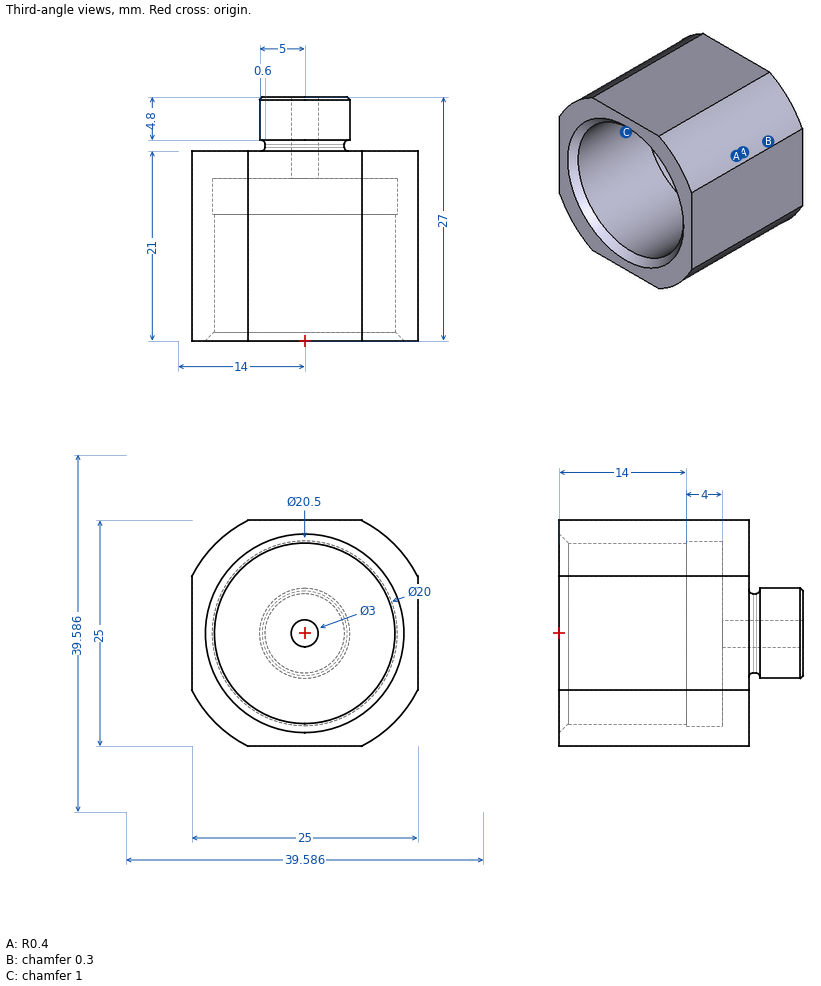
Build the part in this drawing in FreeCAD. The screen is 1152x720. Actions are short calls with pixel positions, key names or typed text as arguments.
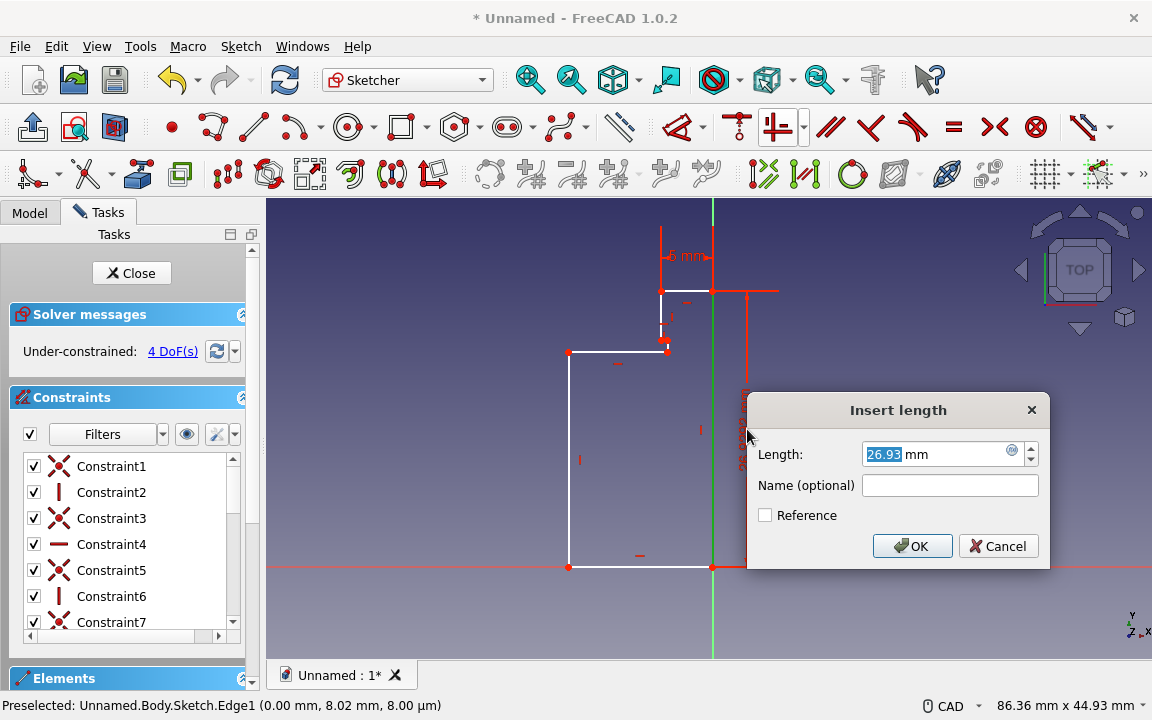
text(27)
key(Return)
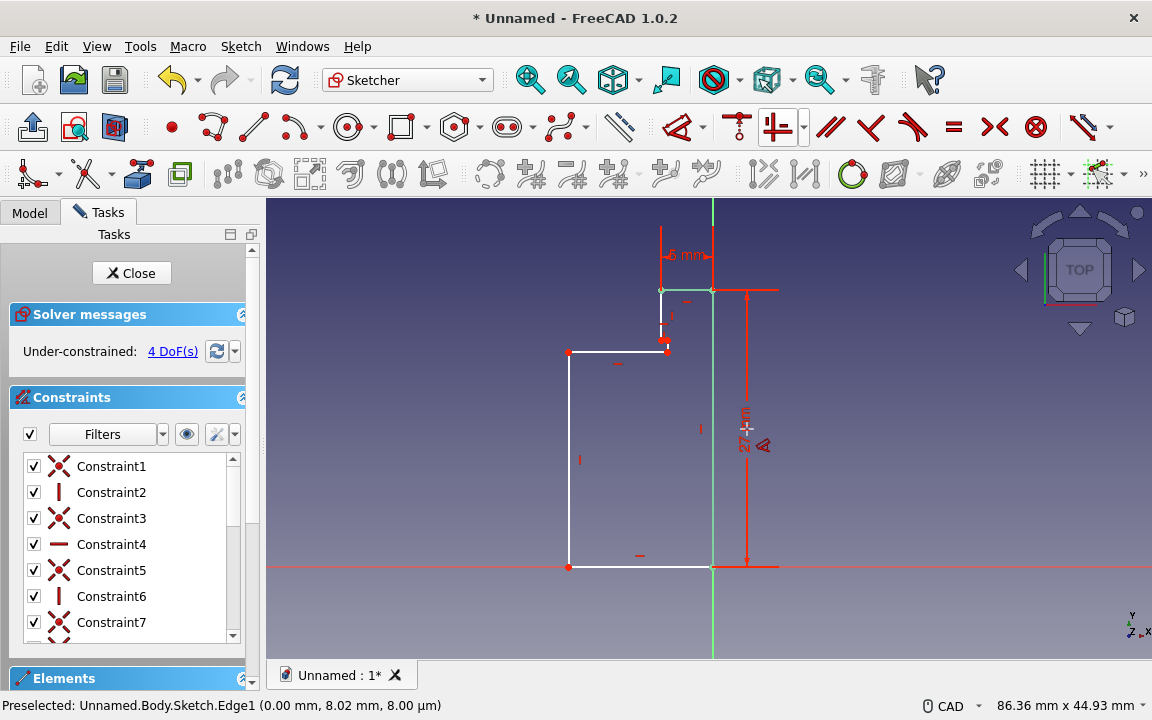
click(569, 417)
click(535, 460)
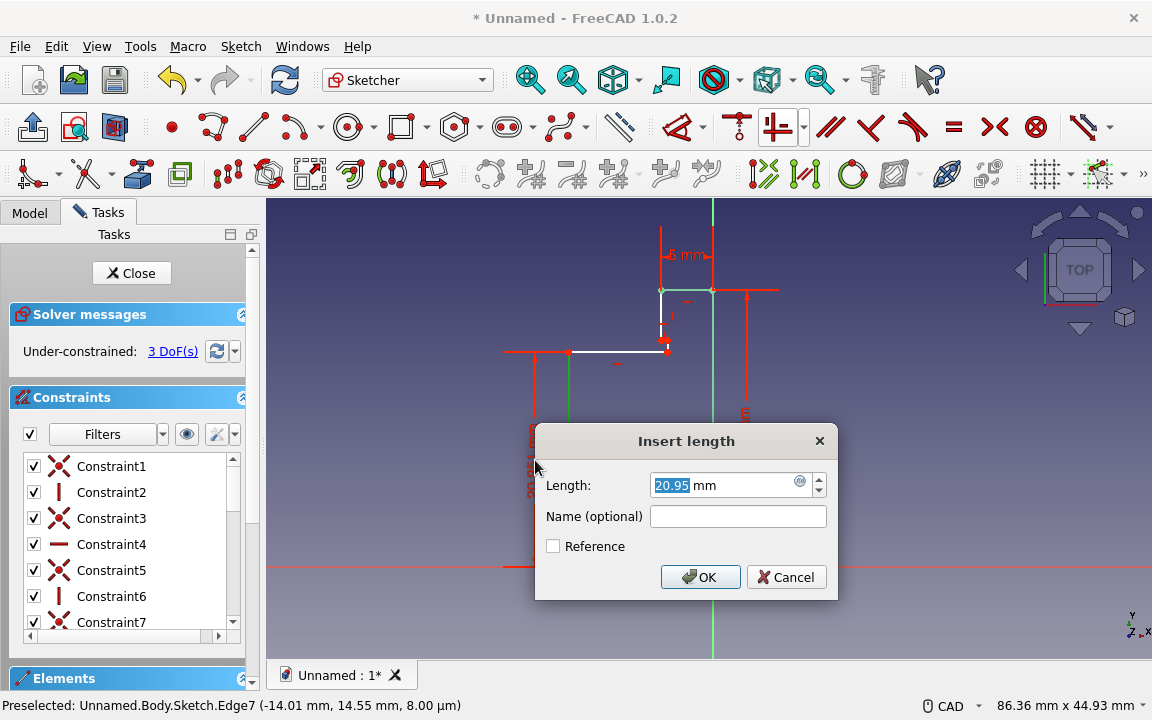
text(21)
key(Return)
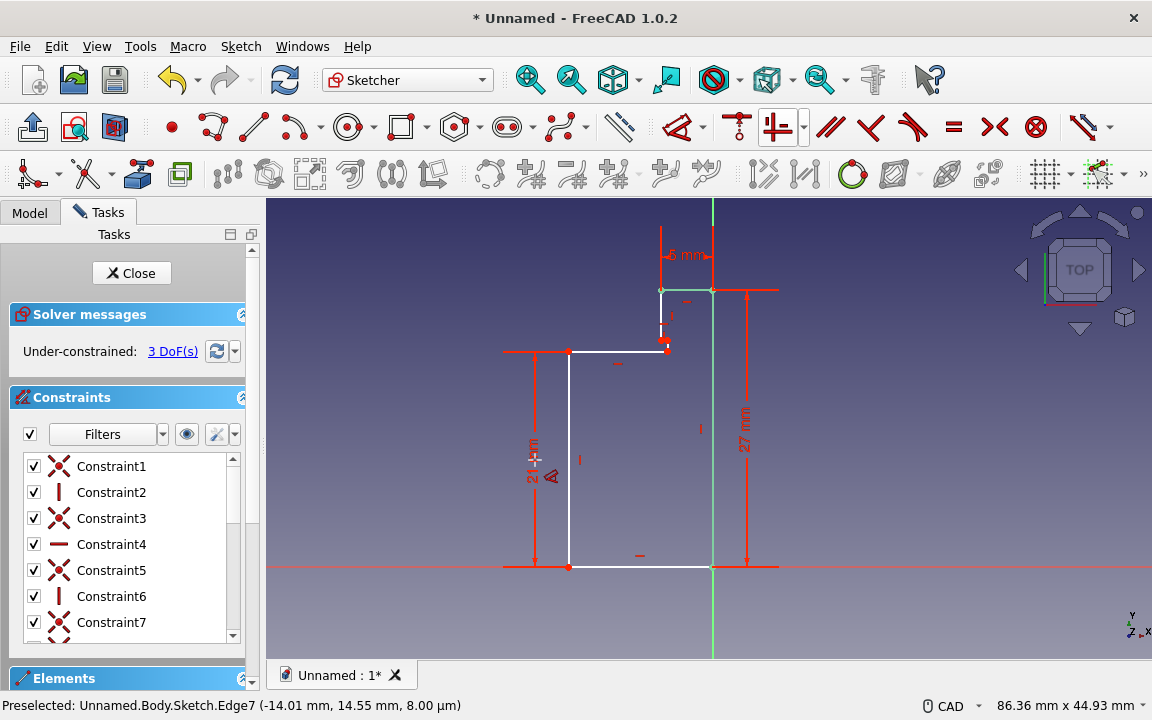
click(612, 567)
click(641, 601)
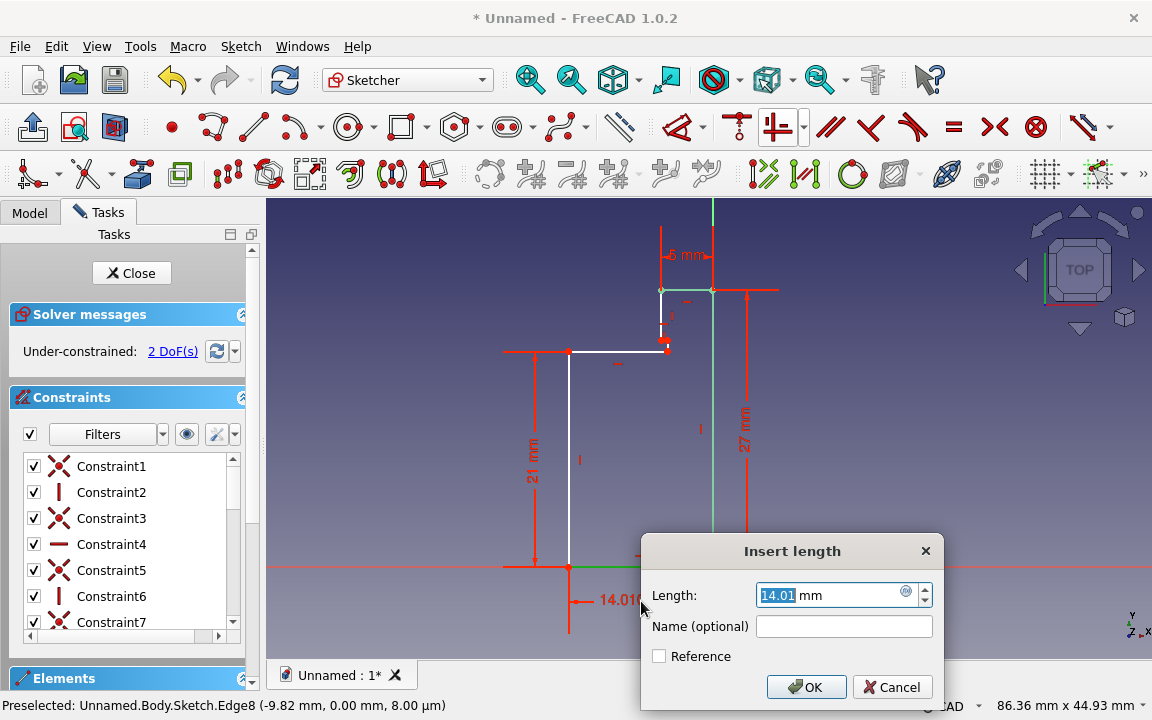
text(14)
key(Return)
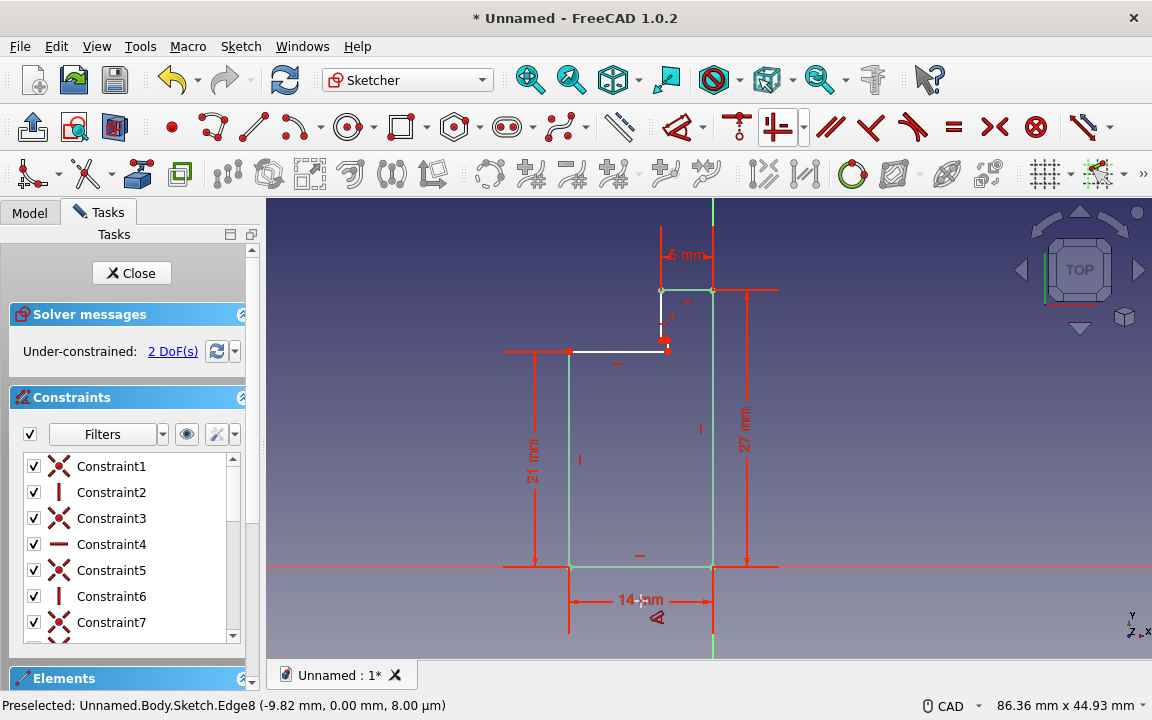
click(661, 305)
click(695, 316)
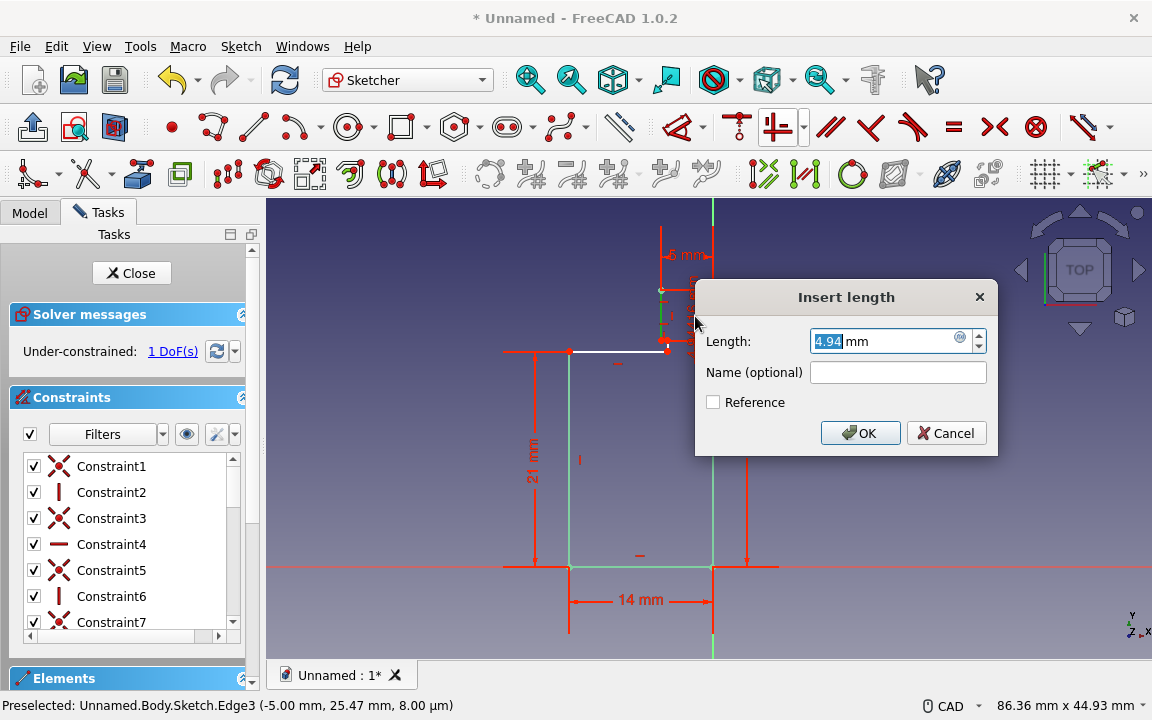
text(4.8)
key(Return)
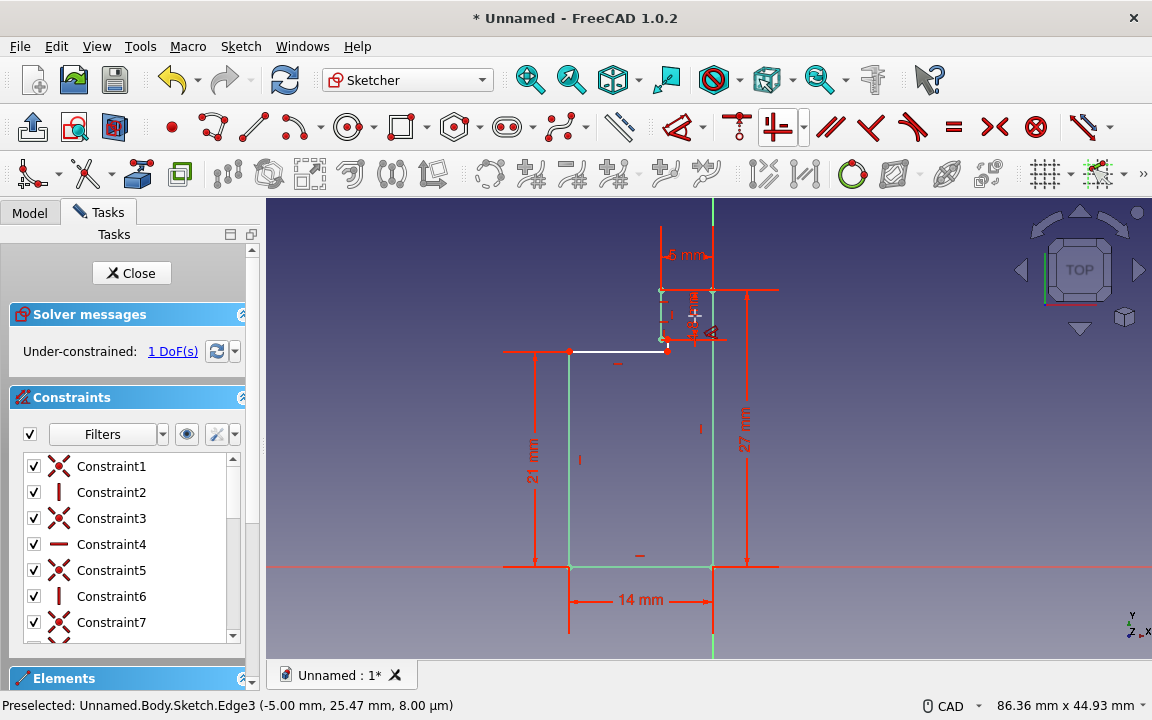
scroll(664, 340, up, 10)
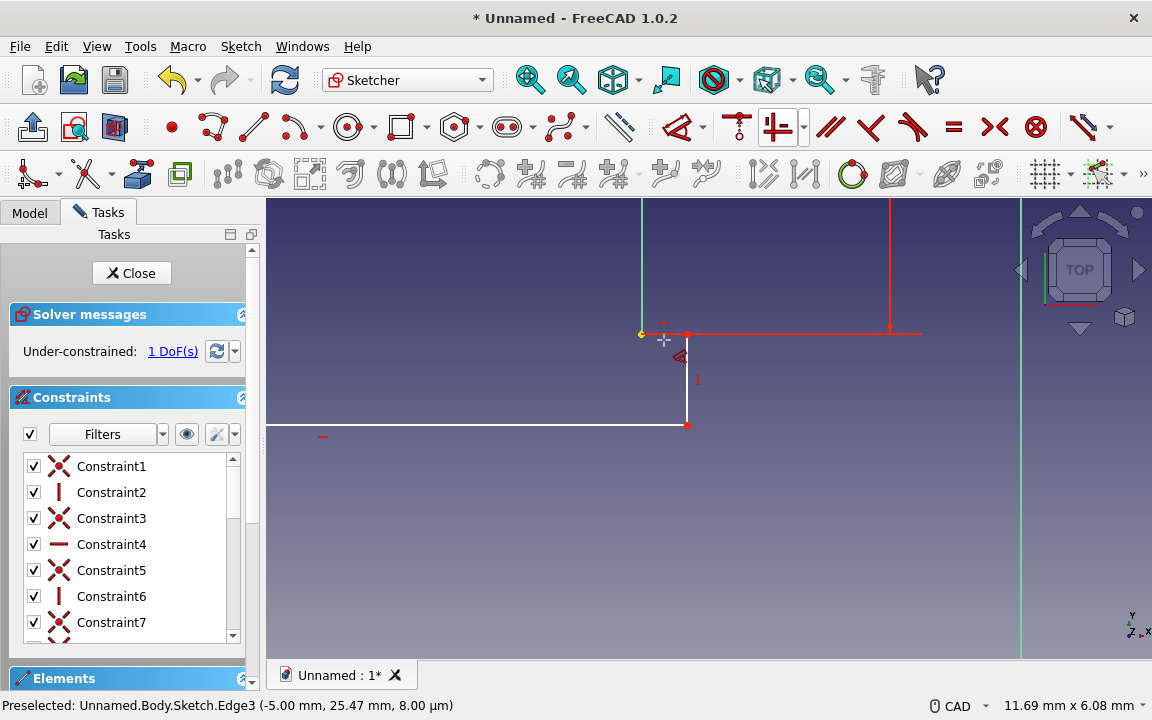
click(665, 334)
click(665, 300)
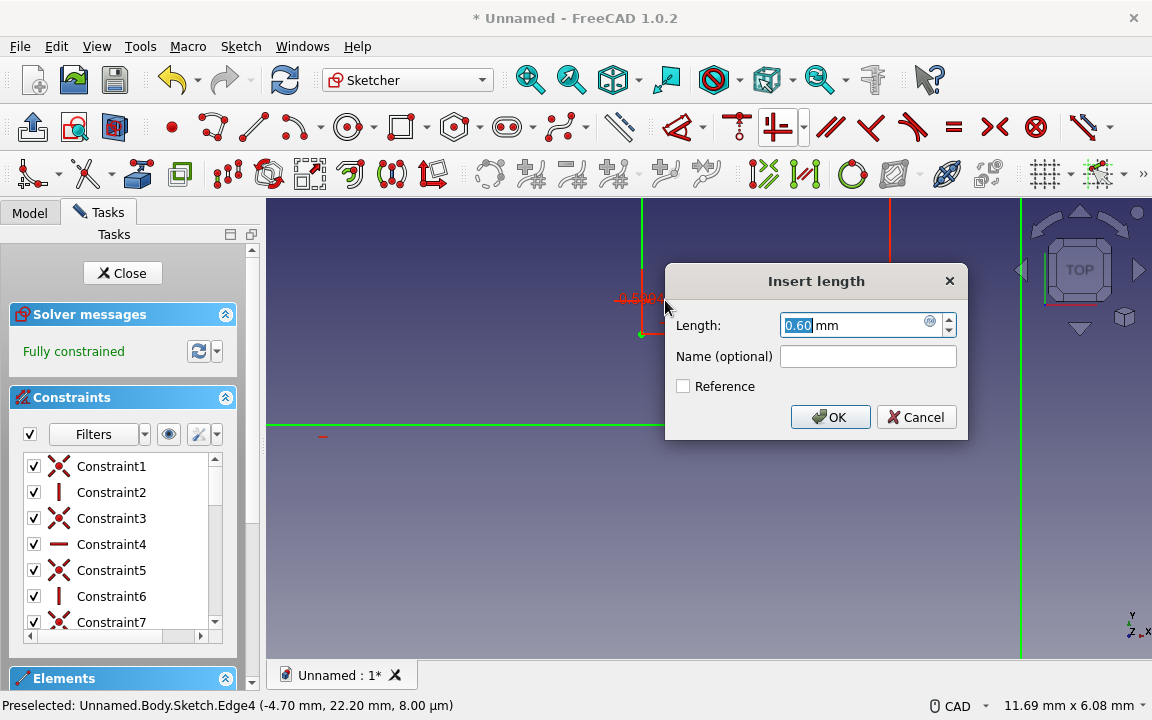
text(0.6)
key(Return)
key(Escape)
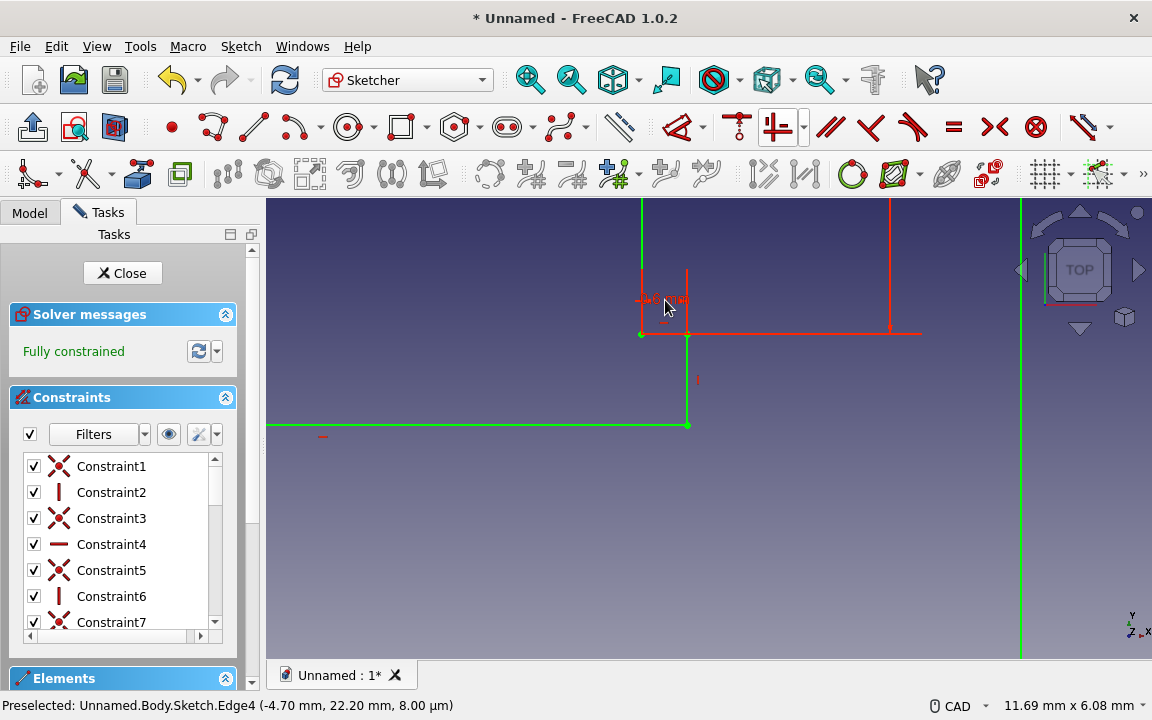
click(123, 273)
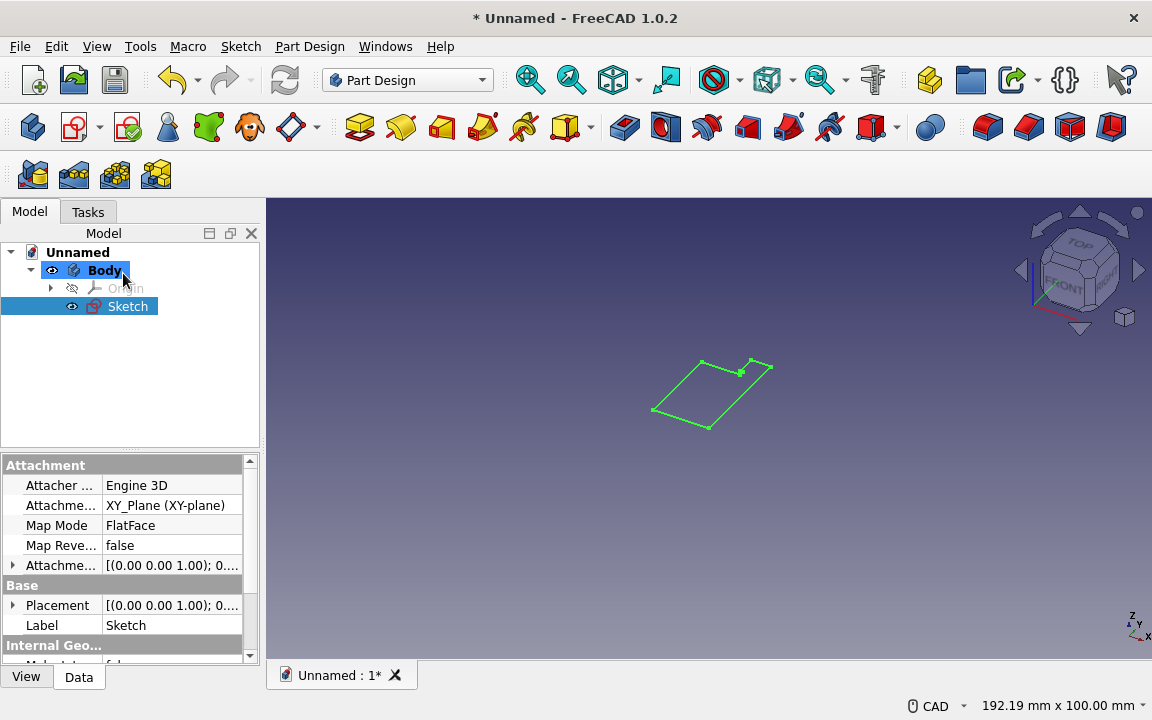
click(401, 128)